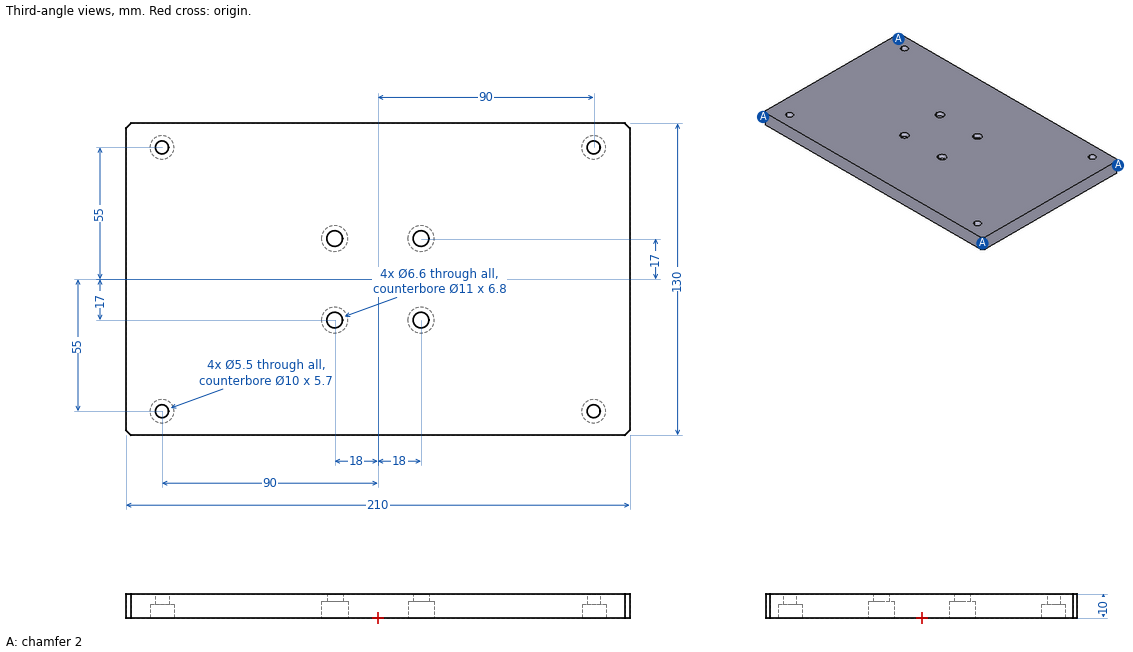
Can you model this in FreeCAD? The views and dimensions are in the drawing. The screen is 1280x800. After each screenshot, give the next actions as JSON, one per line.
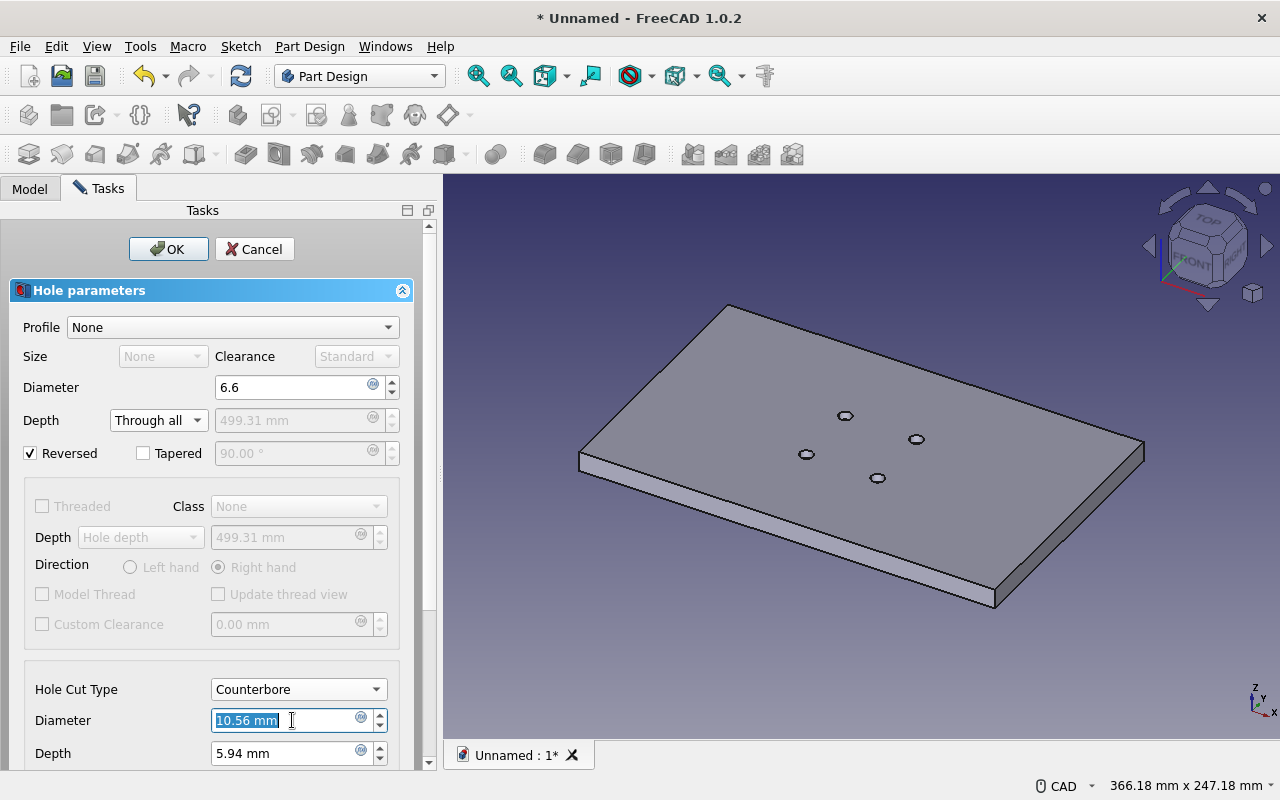
{"action": "type", "text": "11"}
{"action": "key", "text": "Tab"}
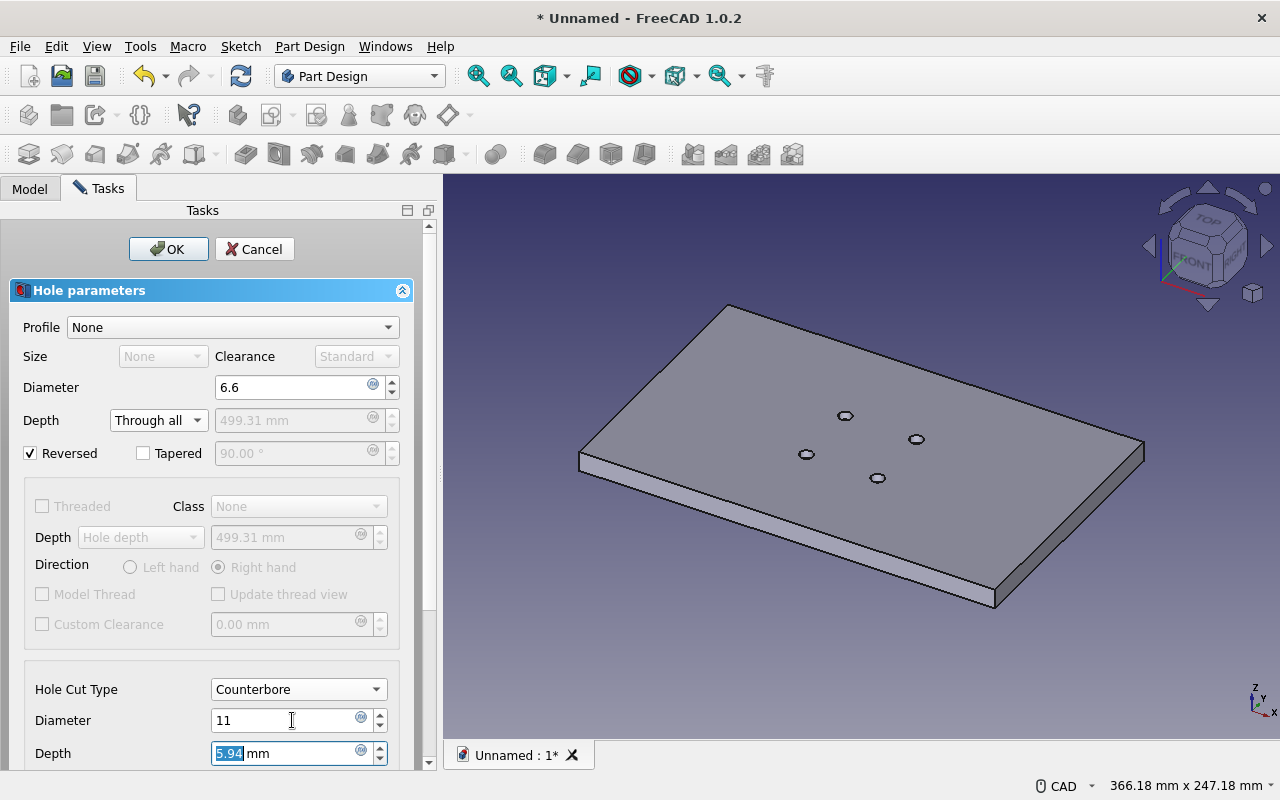
{"action": "type", "text": "6.8"}
{"action": "key", "text": "Tab"}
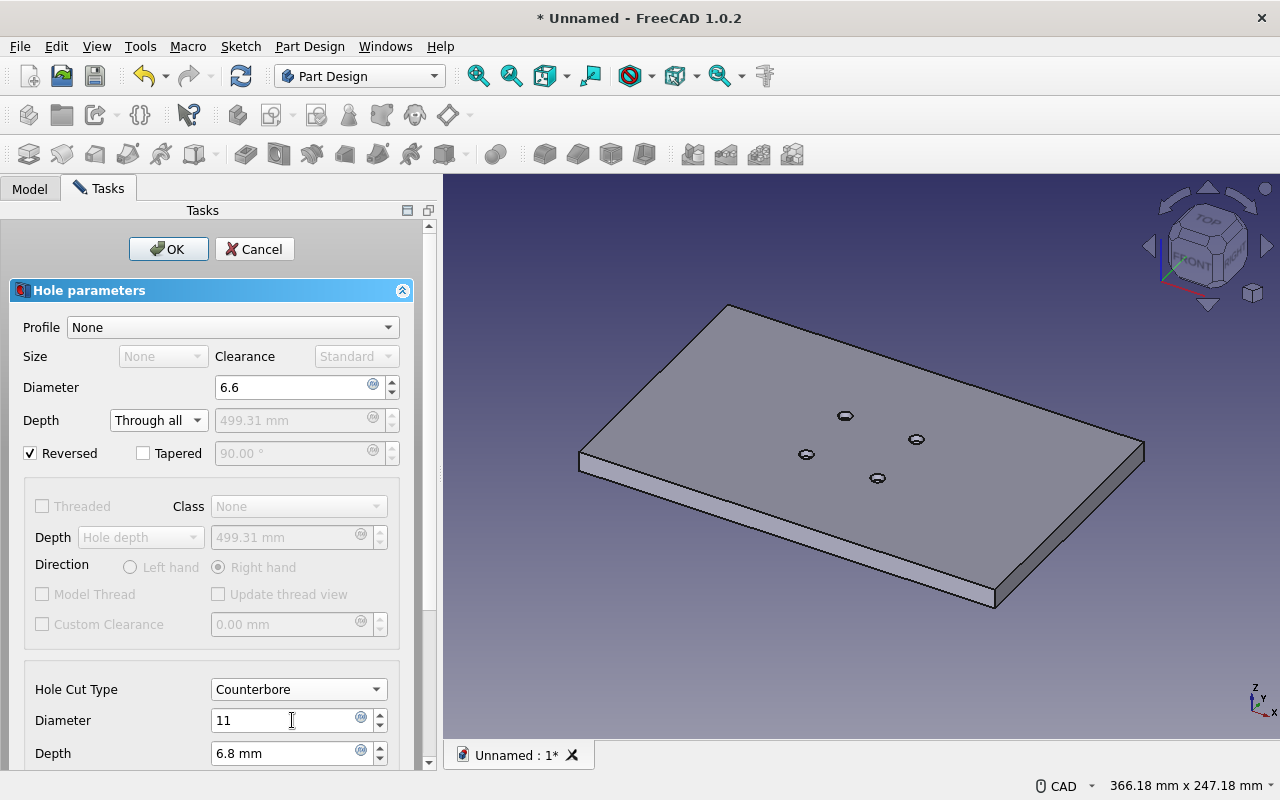
{"action": "left_click", "coordinate": [169, 249]}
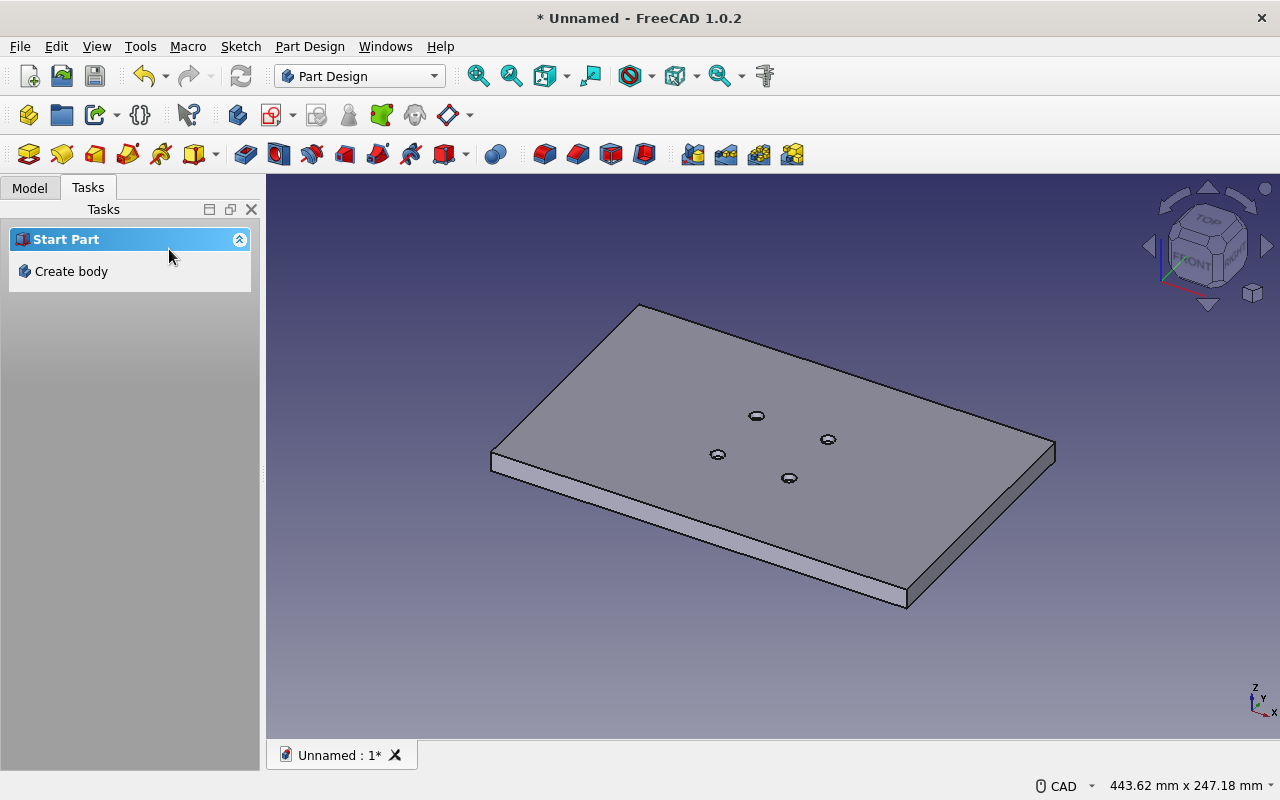
{"action": "key", "text": "5"}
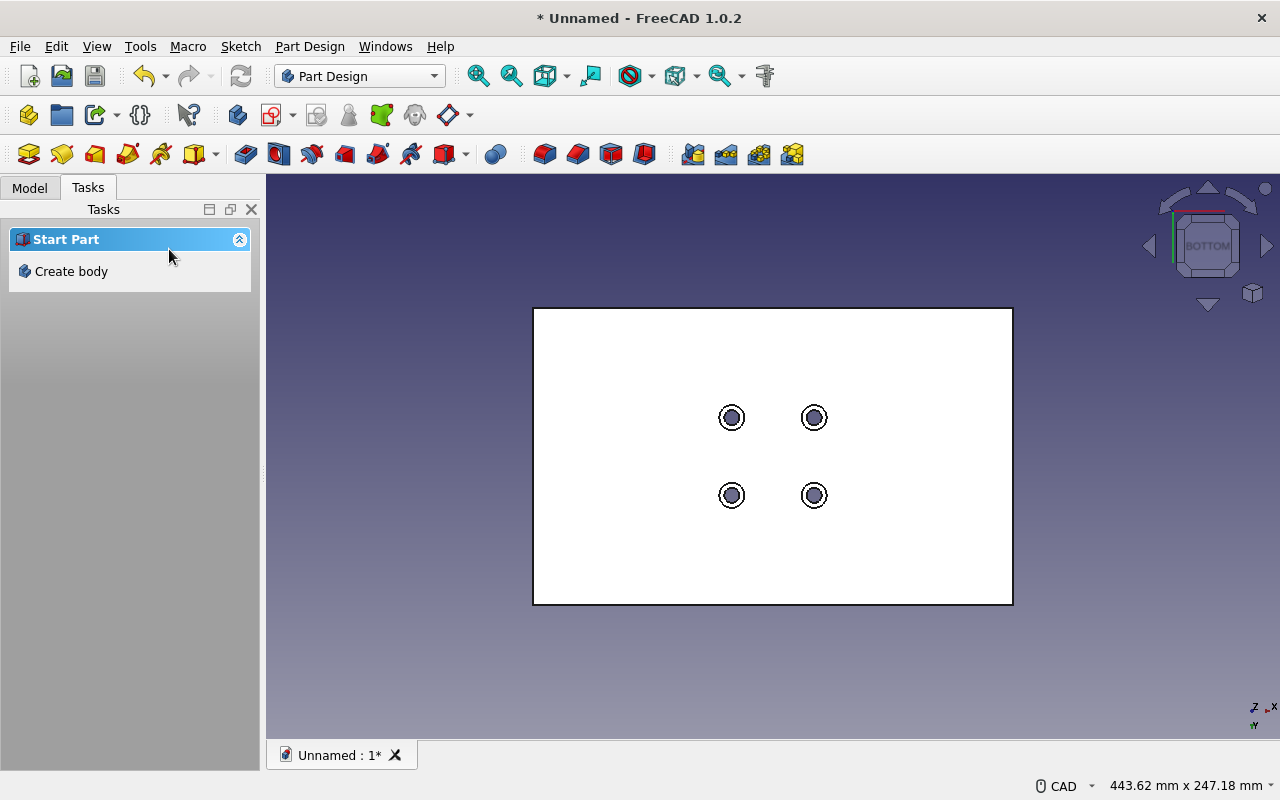
{"action": "left_click", "coordinate": [636, 455]}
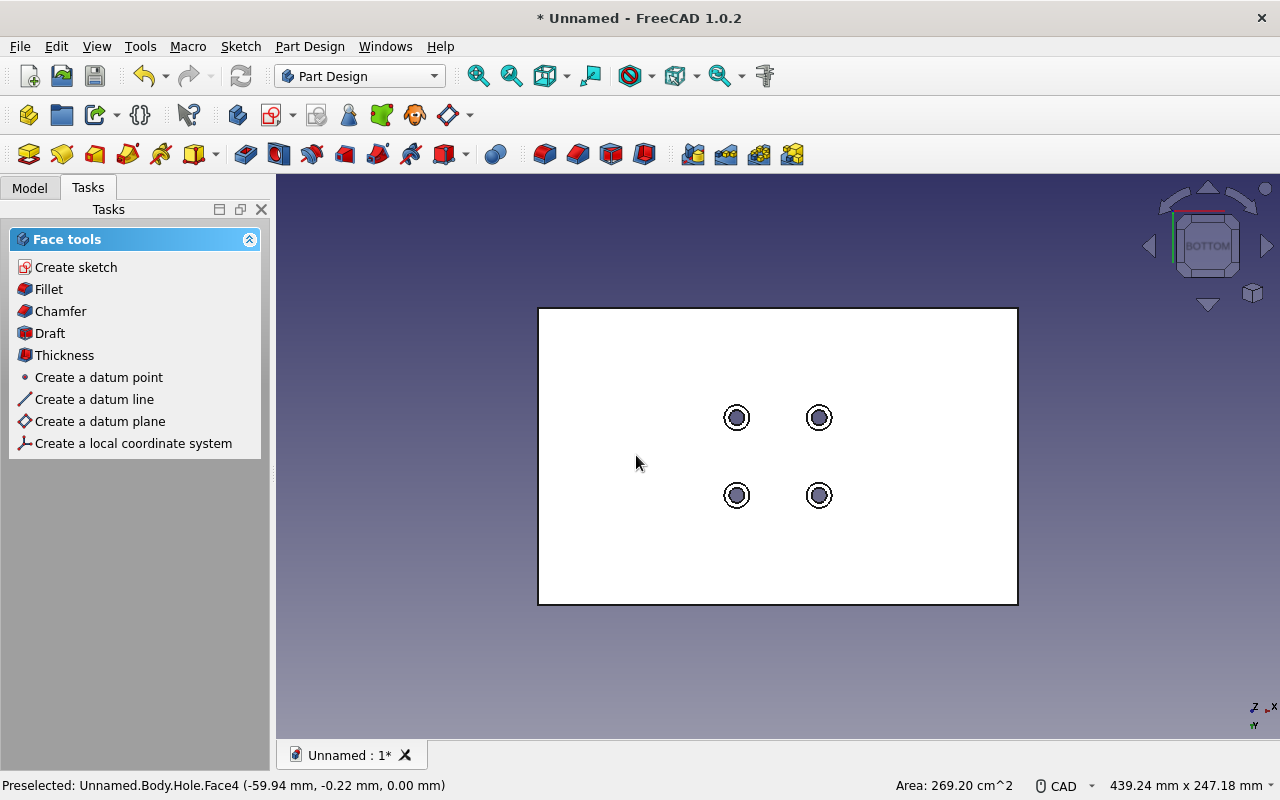
{"action": "left_click", "coordinate": [270, 116]}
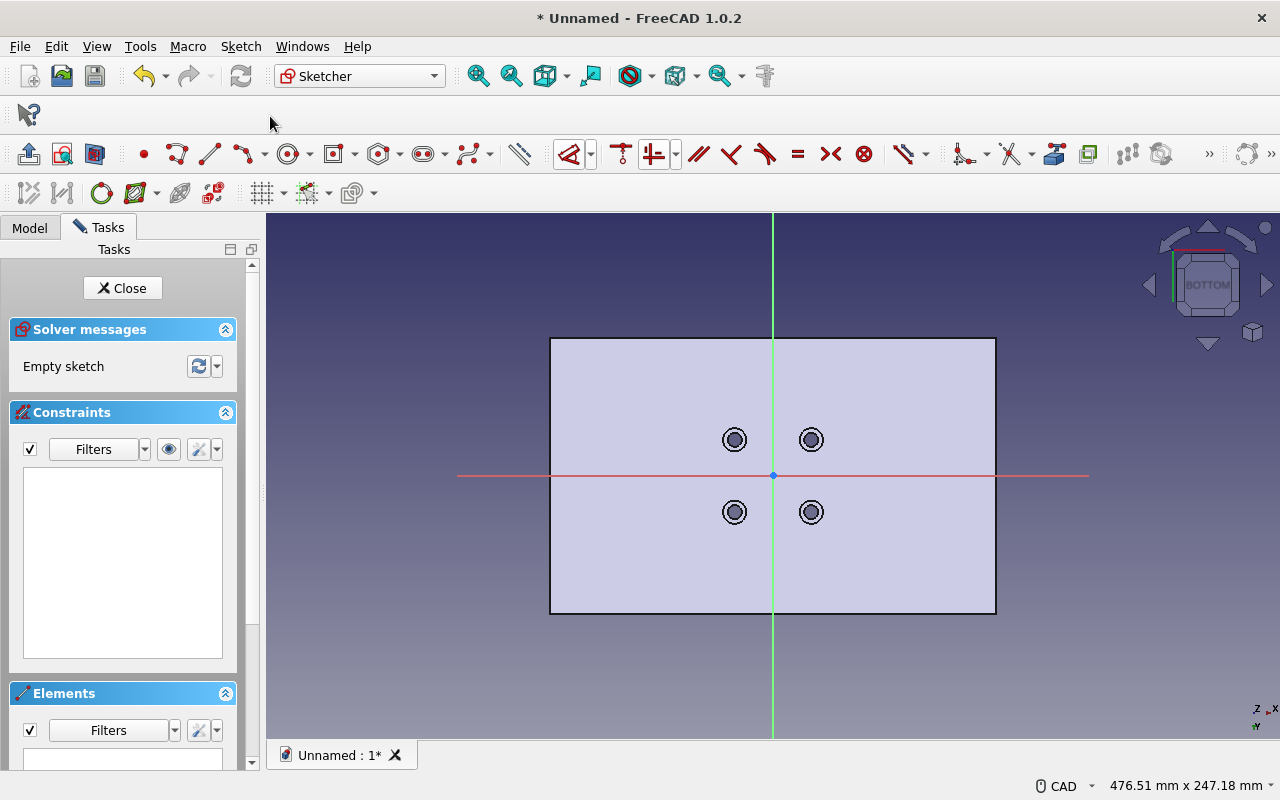
{"action": "left_click", "coordinate": [288, 154]}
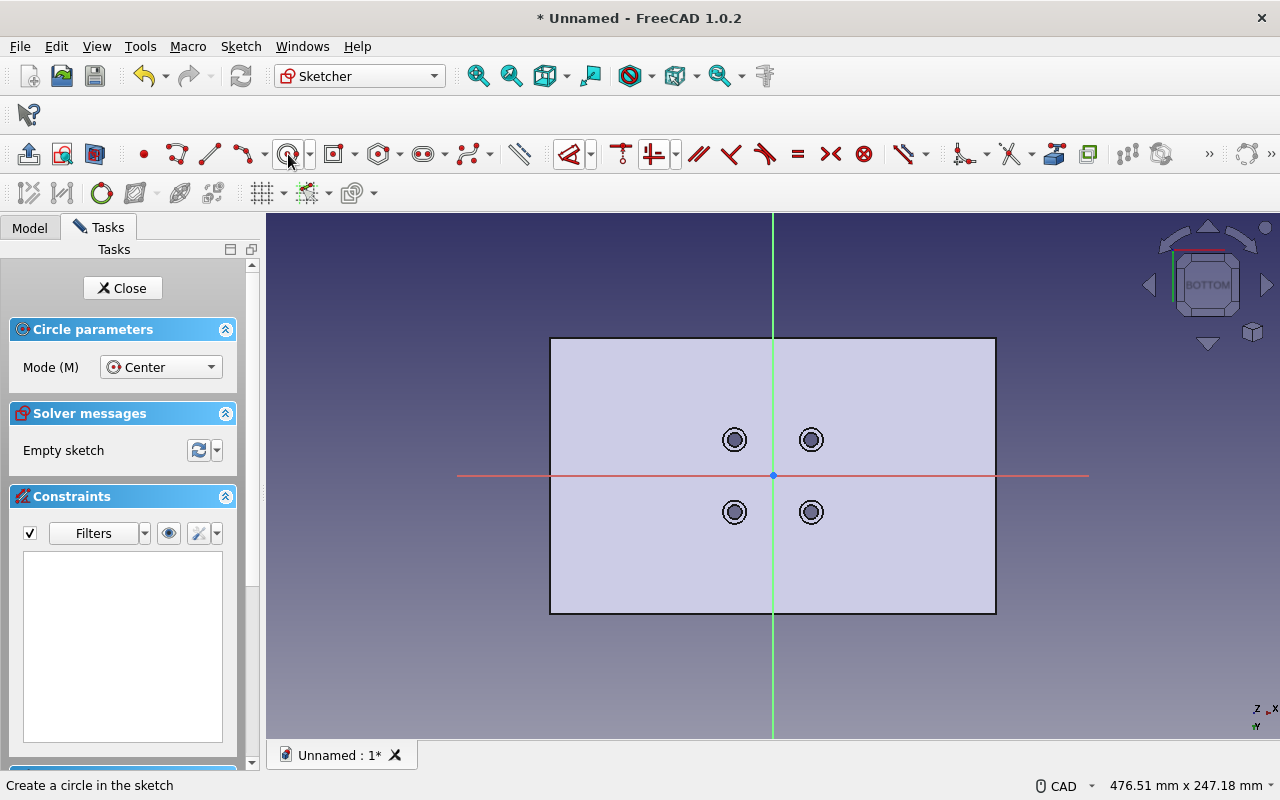
{"action": "scroll", "coordinate": [581, 359], "scroll_direction": "up", "scroll_amount": 7}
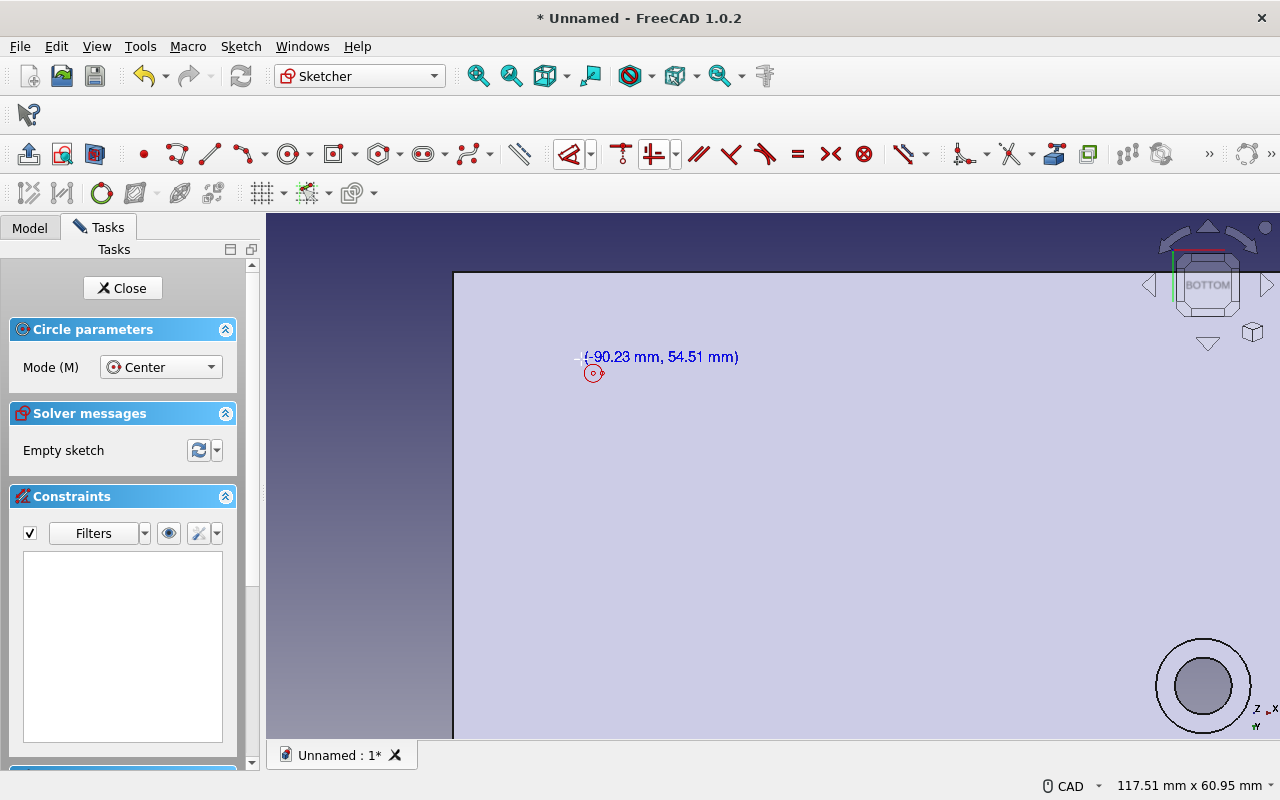
{"action": "scroll", "coordinate": [423, 322], "scroll_direction": "down", "scroll_amount": 6}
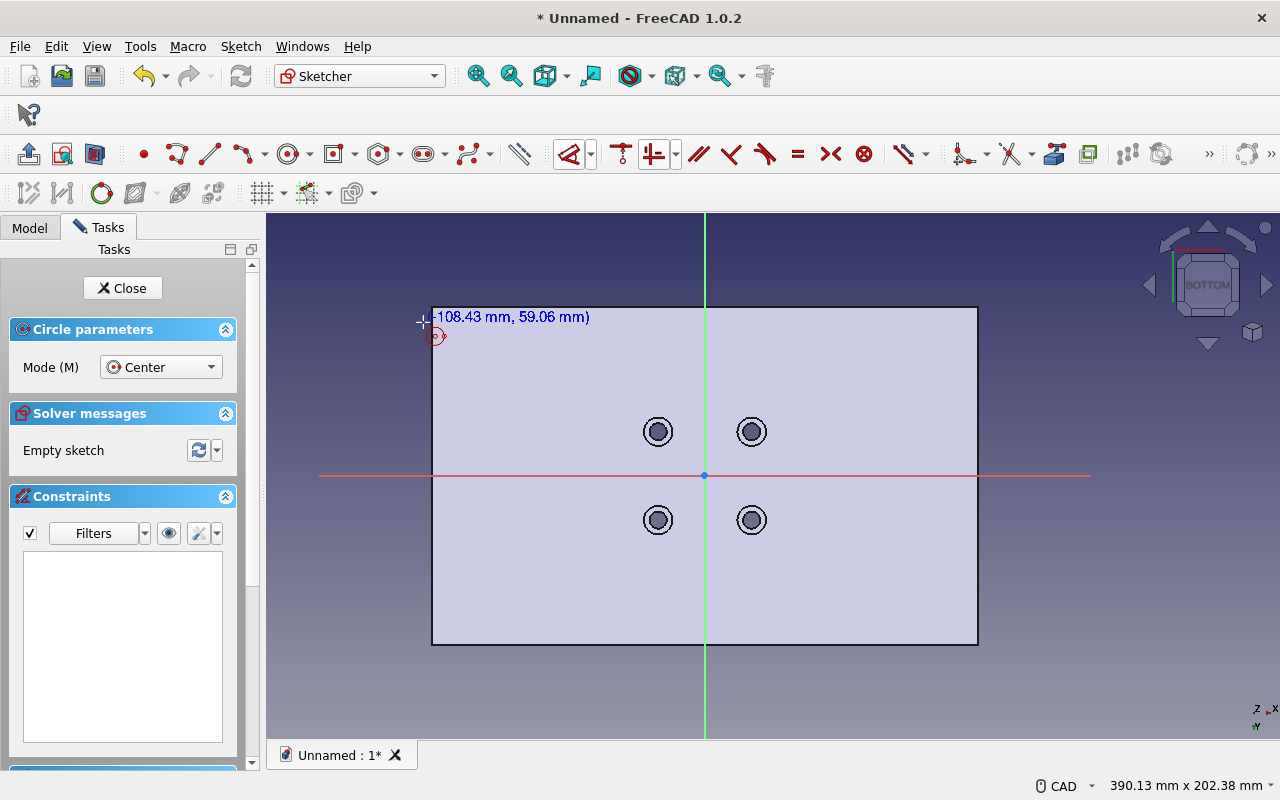
{"action": "left_click", "coordinate": [471, 333]}
{"action": "mouse_move", "coordinate": [476, 328]}